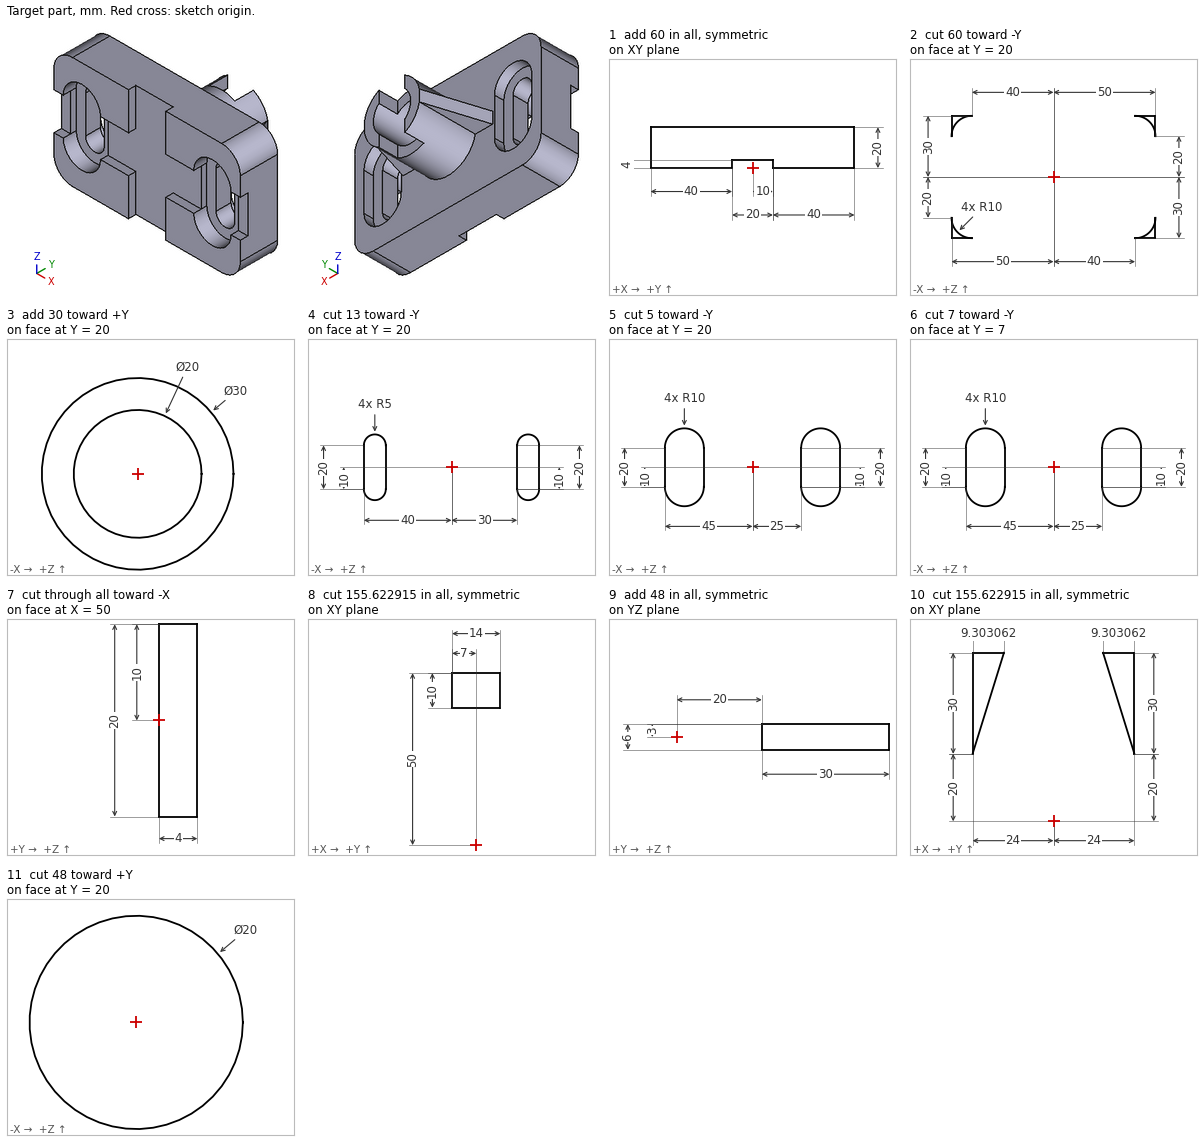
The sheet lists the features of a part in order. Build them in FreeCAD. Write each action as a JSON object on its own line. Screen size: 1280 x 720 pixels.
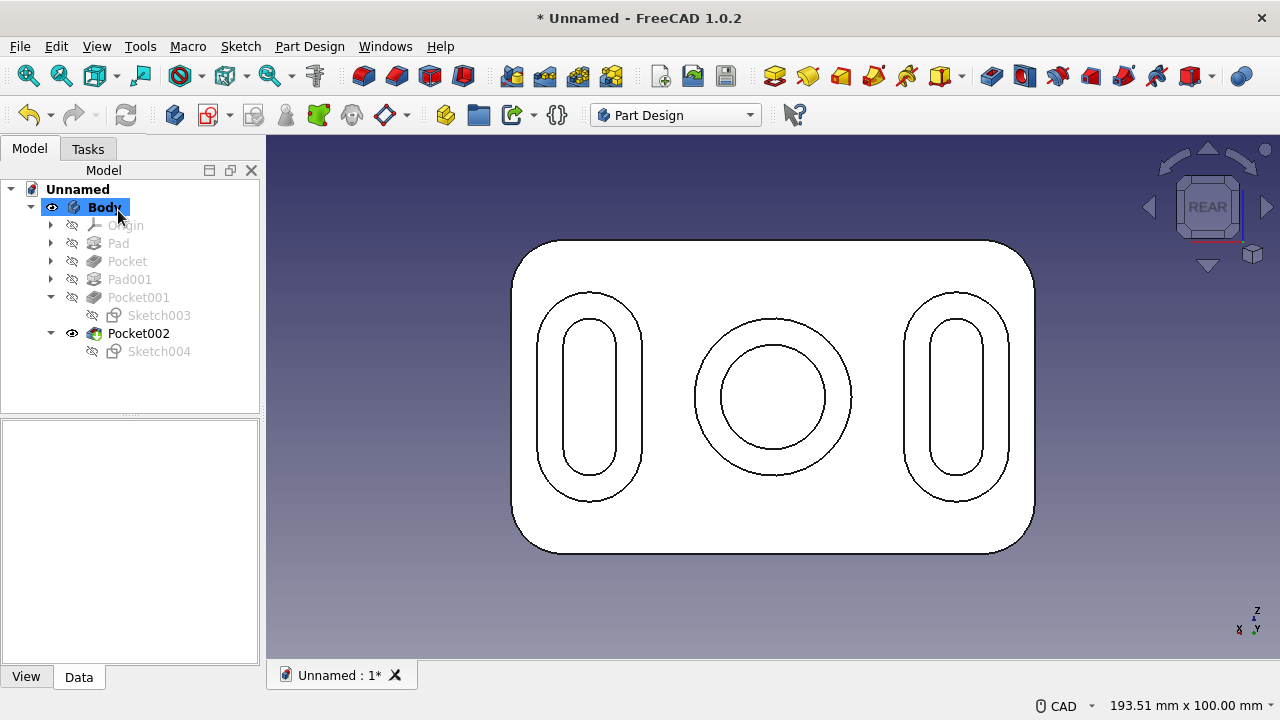
{"action": "left_click", "coordinate": [590, 351]}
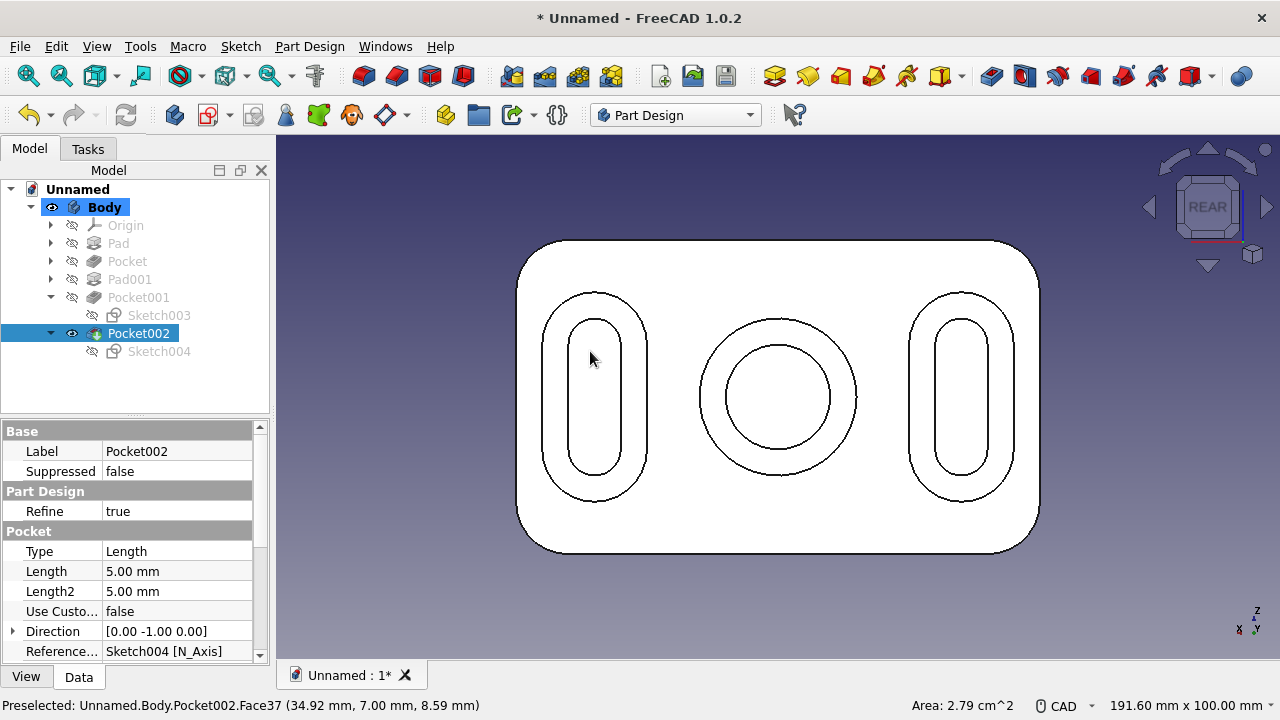
{"action": "left_click", "coordinate": [208, 116]}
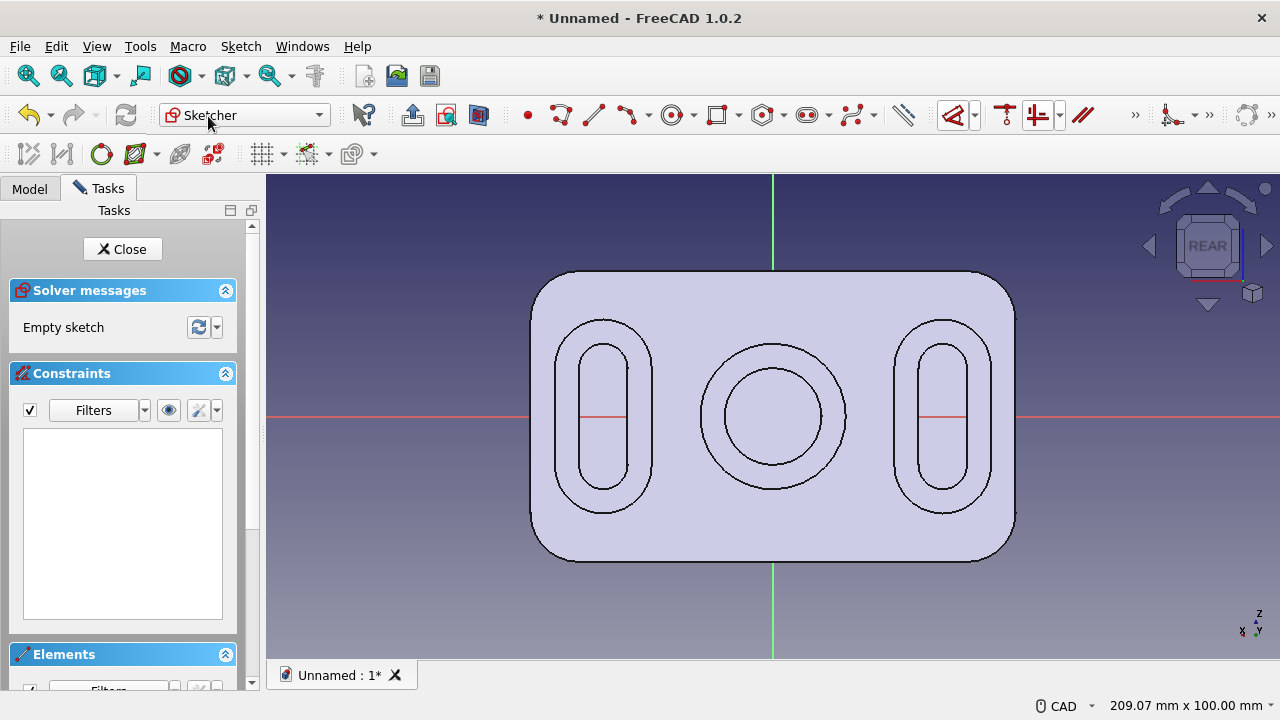
{"action": "left_click", "coordinate": [806, 116]}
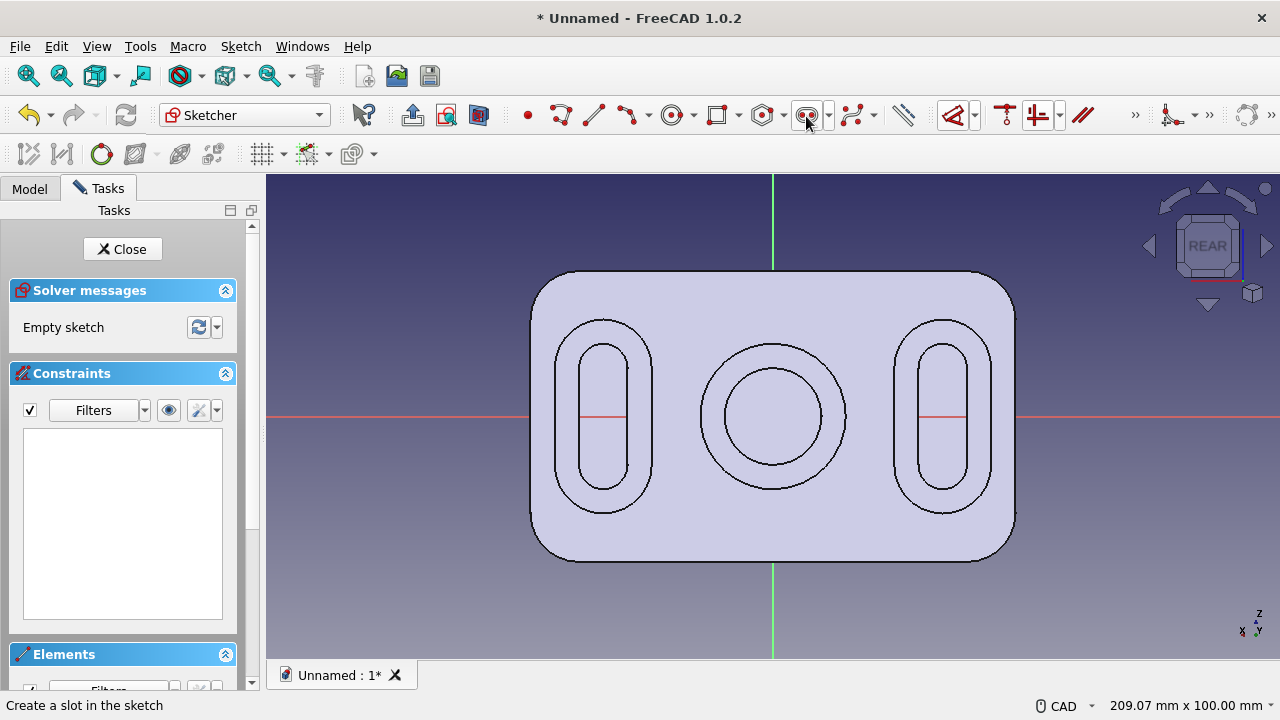
{"action": "left_click", "coordinate": [603, 465]}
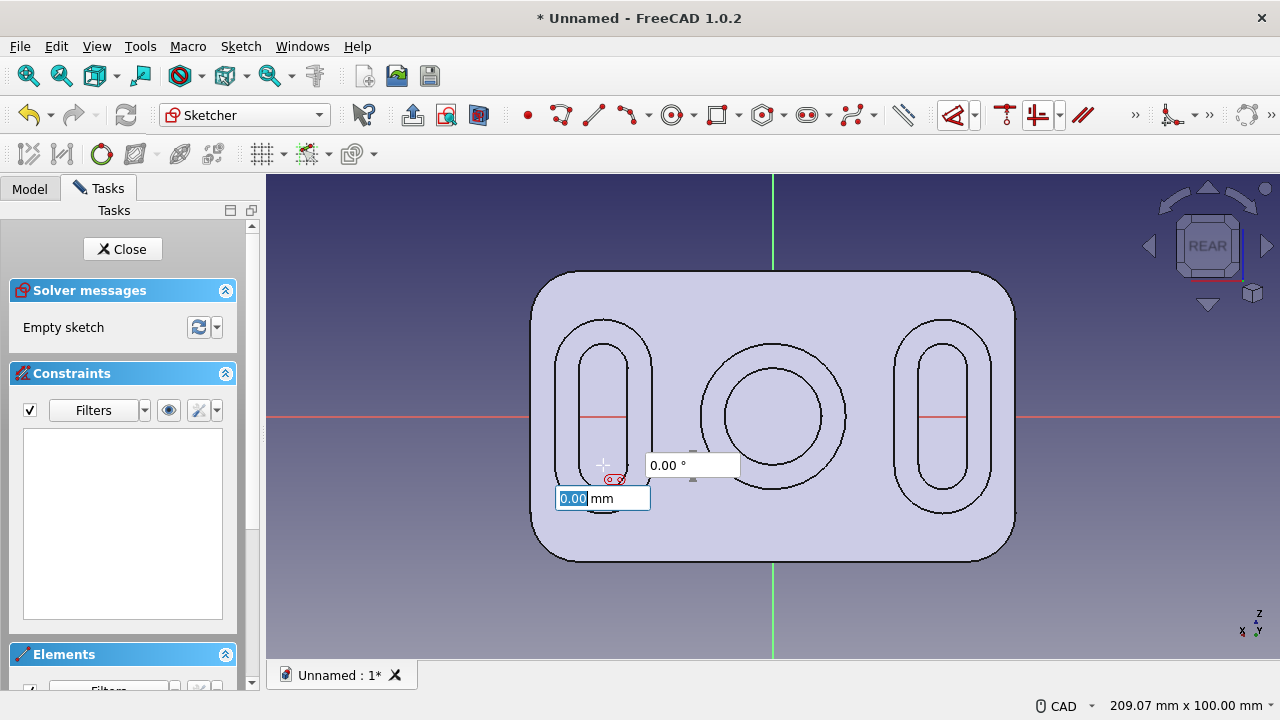
{"action": "left_click", "coordinate": [603, 368]}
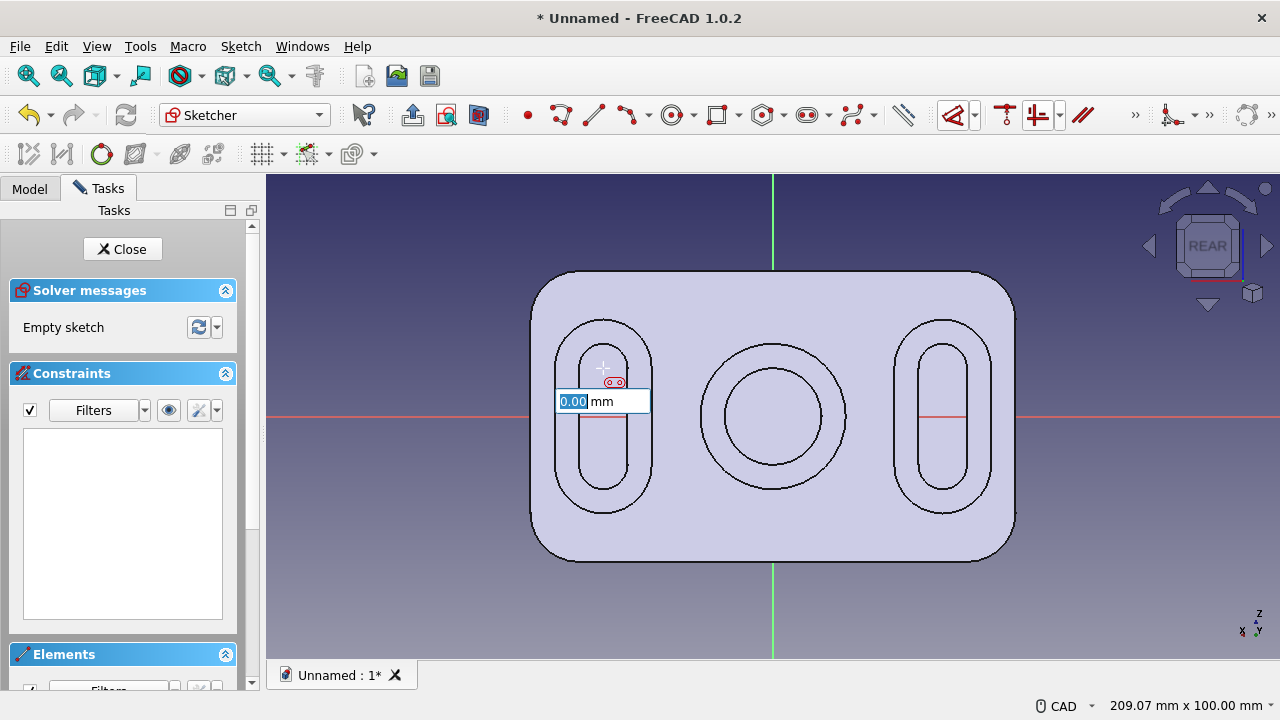
{"action": "left_click", "coordinate": [555, 431]}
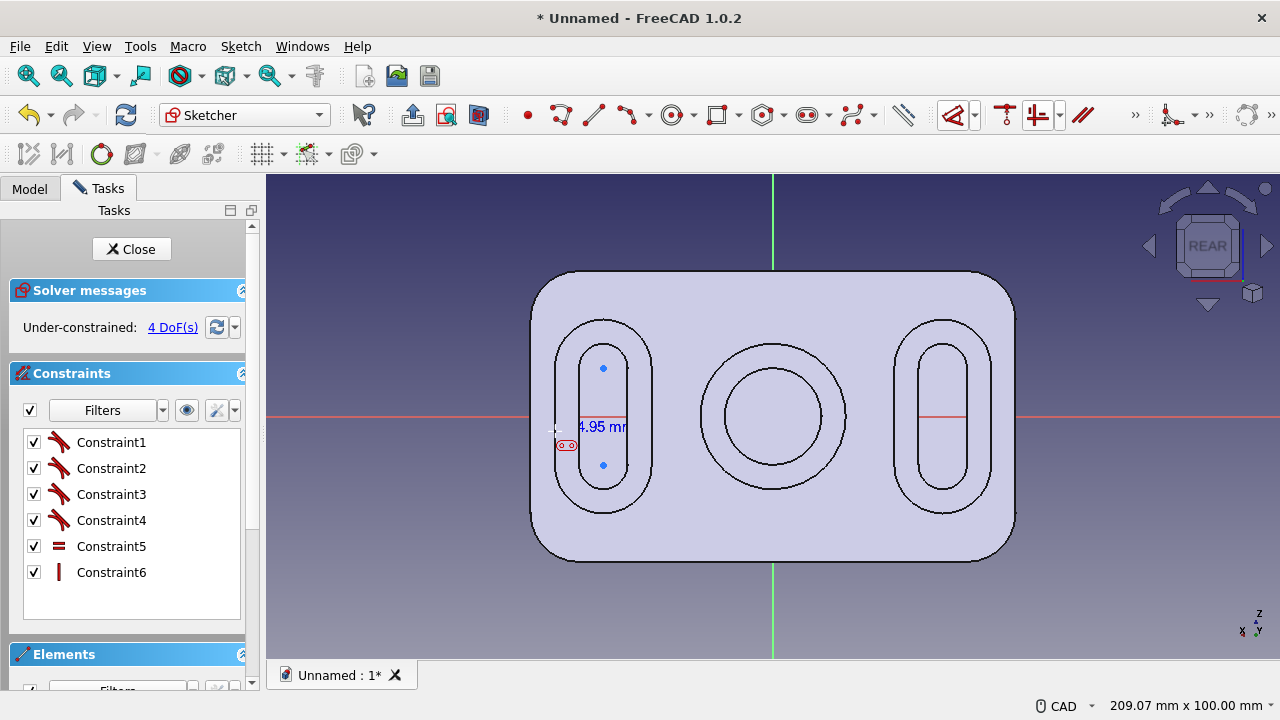
{"action": "left_click", "coordinate": [943, 465]}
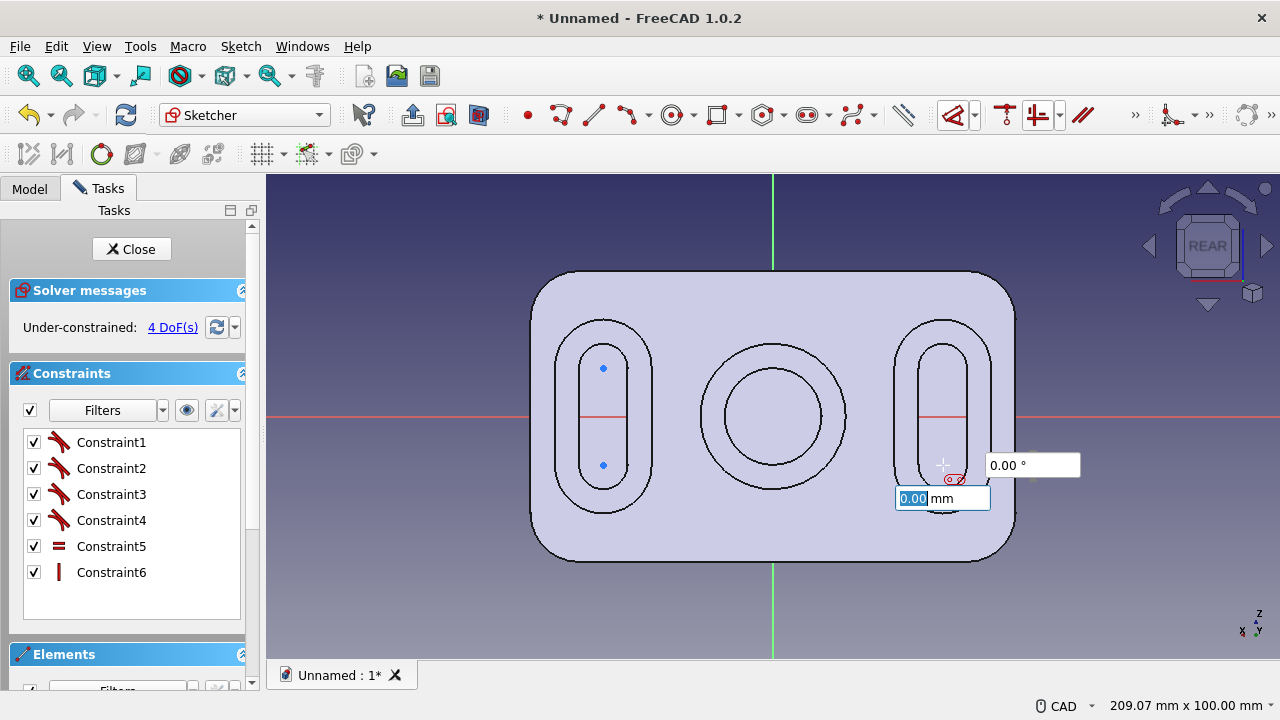
{"action": "left_click", "coordinate": [943, 368]}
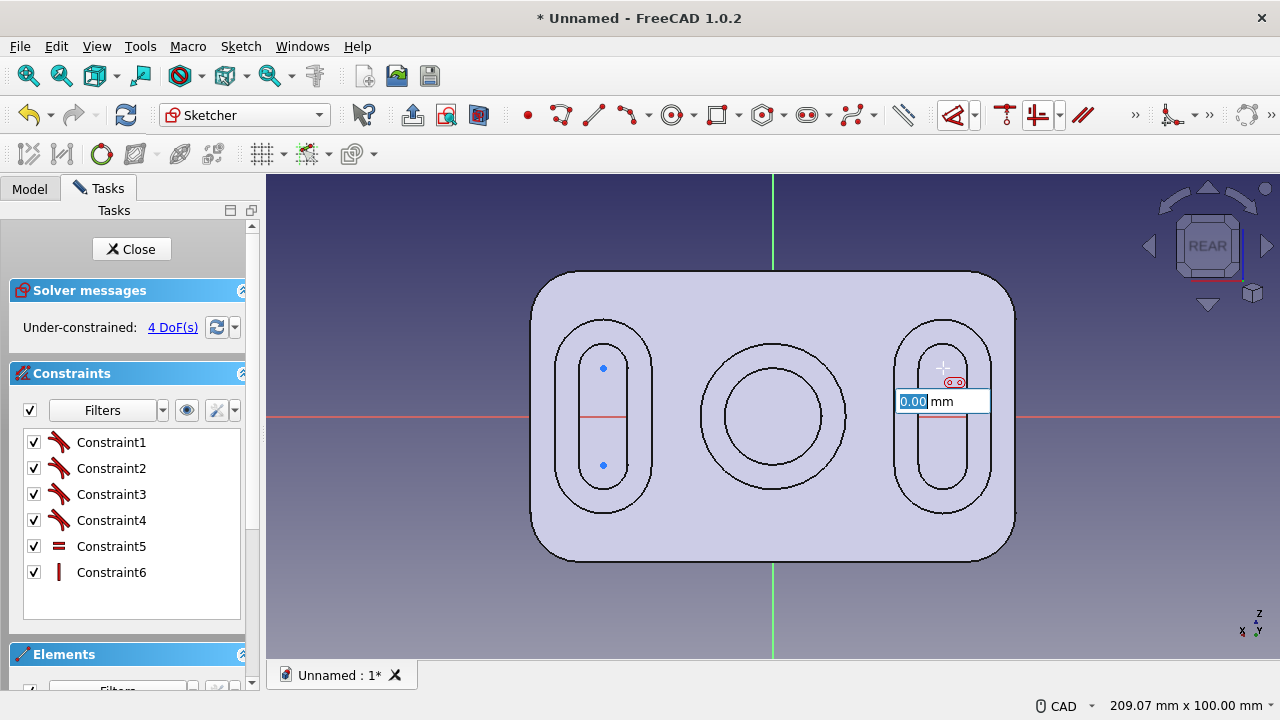
{"action": "left_click", "coordinate": [991, 402]}
{"action": "key", "text": "Escape"}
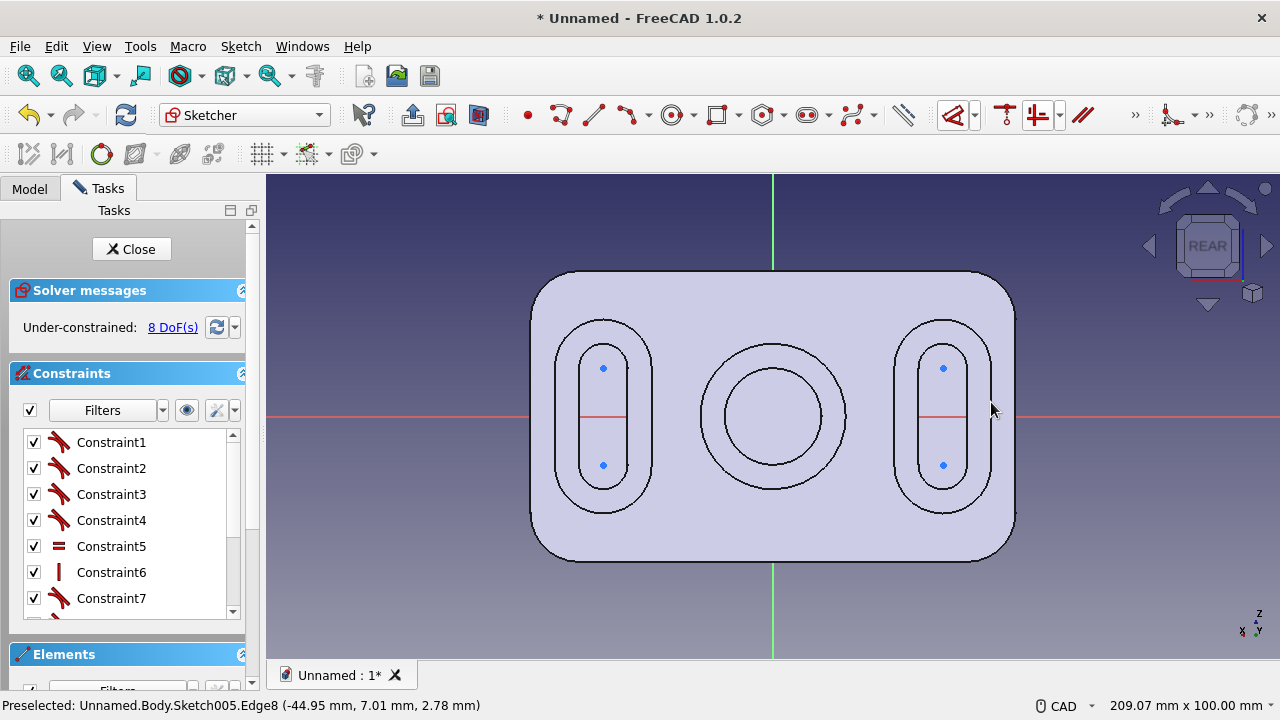
{"action": "left_click", "coordinate": [575, 505]}